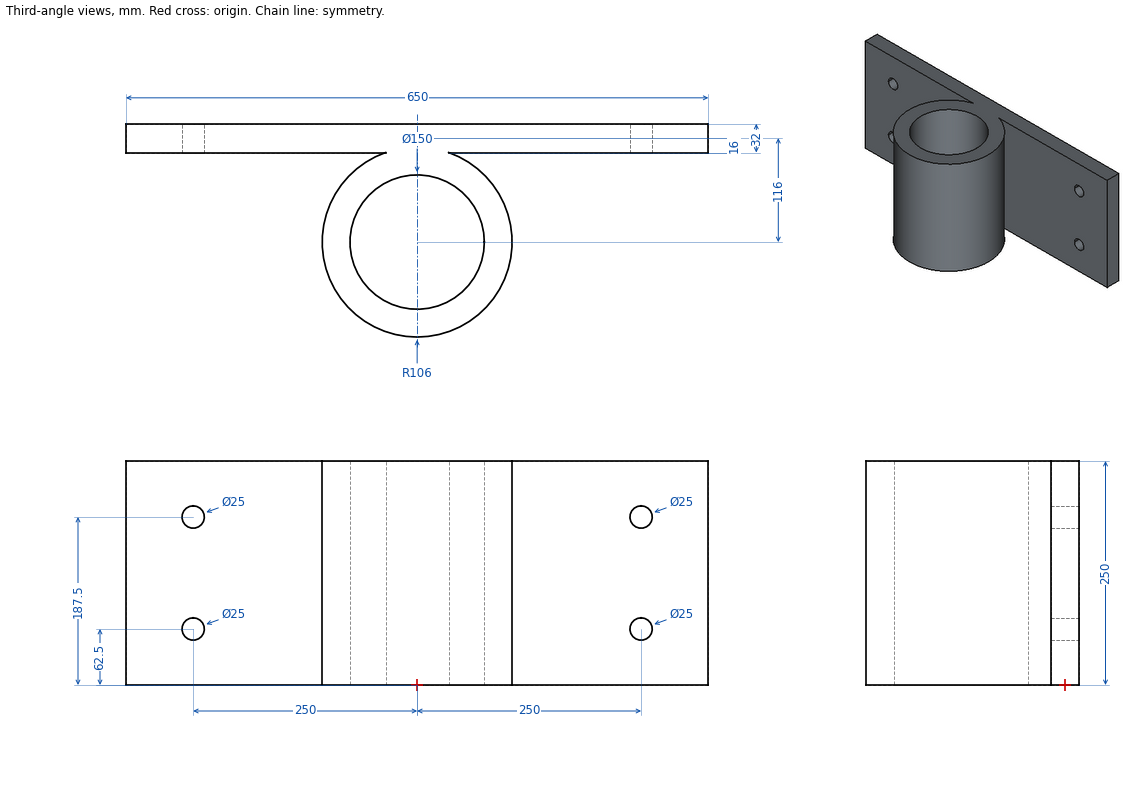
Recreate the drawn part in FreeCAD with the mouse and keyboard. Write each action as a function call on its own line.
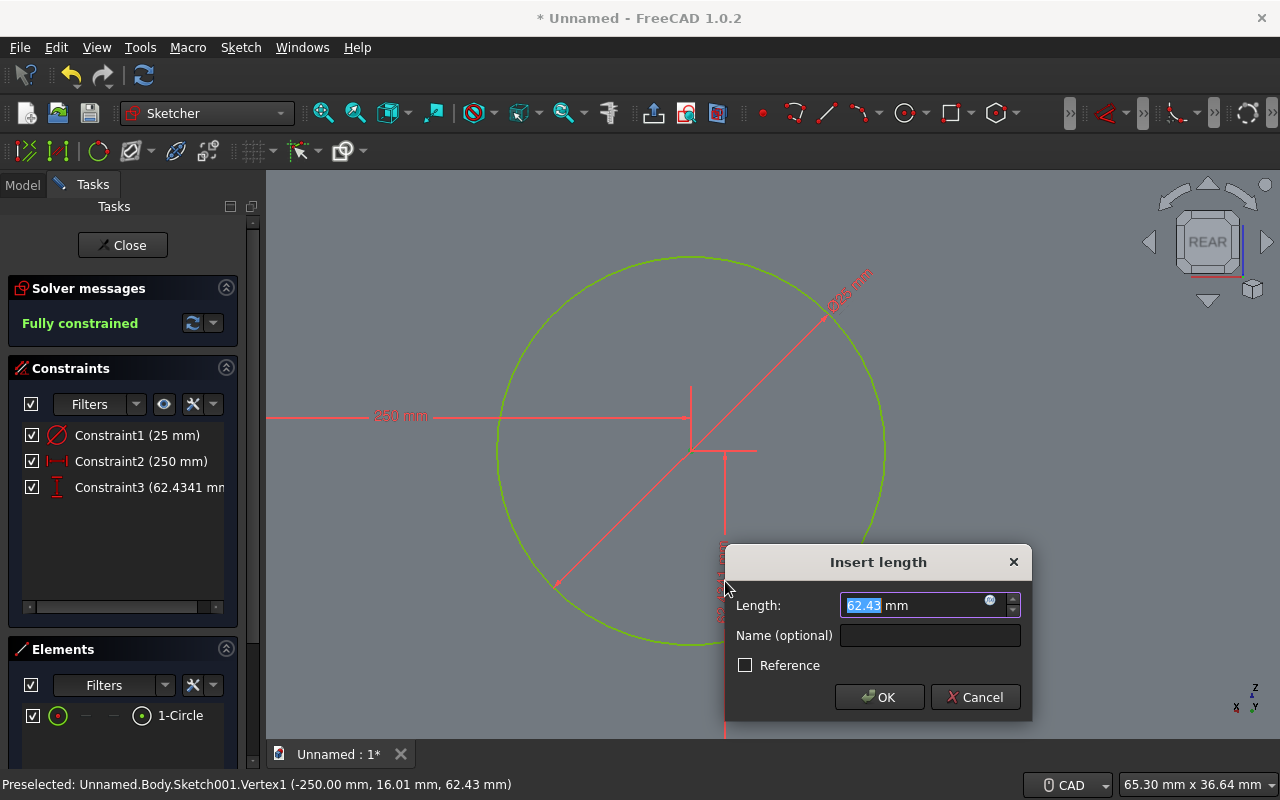
text(62.5)
key(Return)
key(Escape)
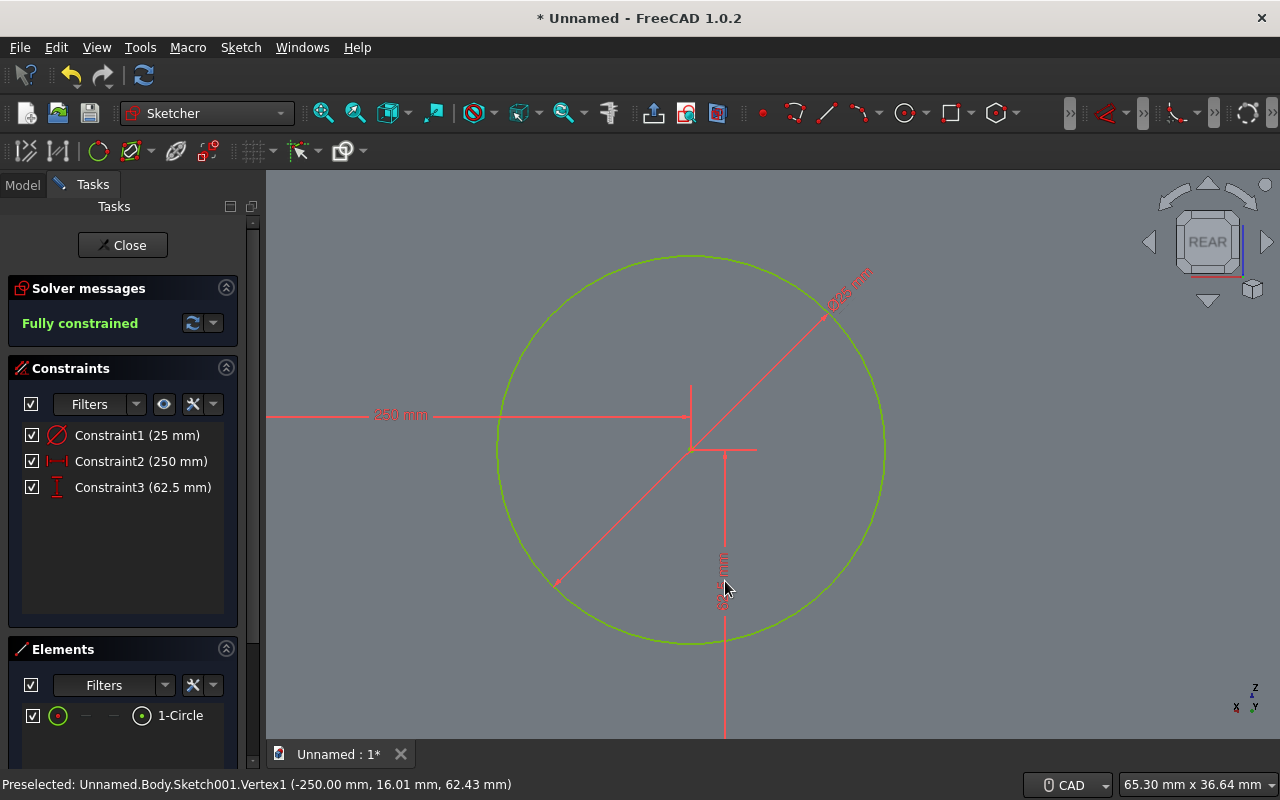
click(123, 245)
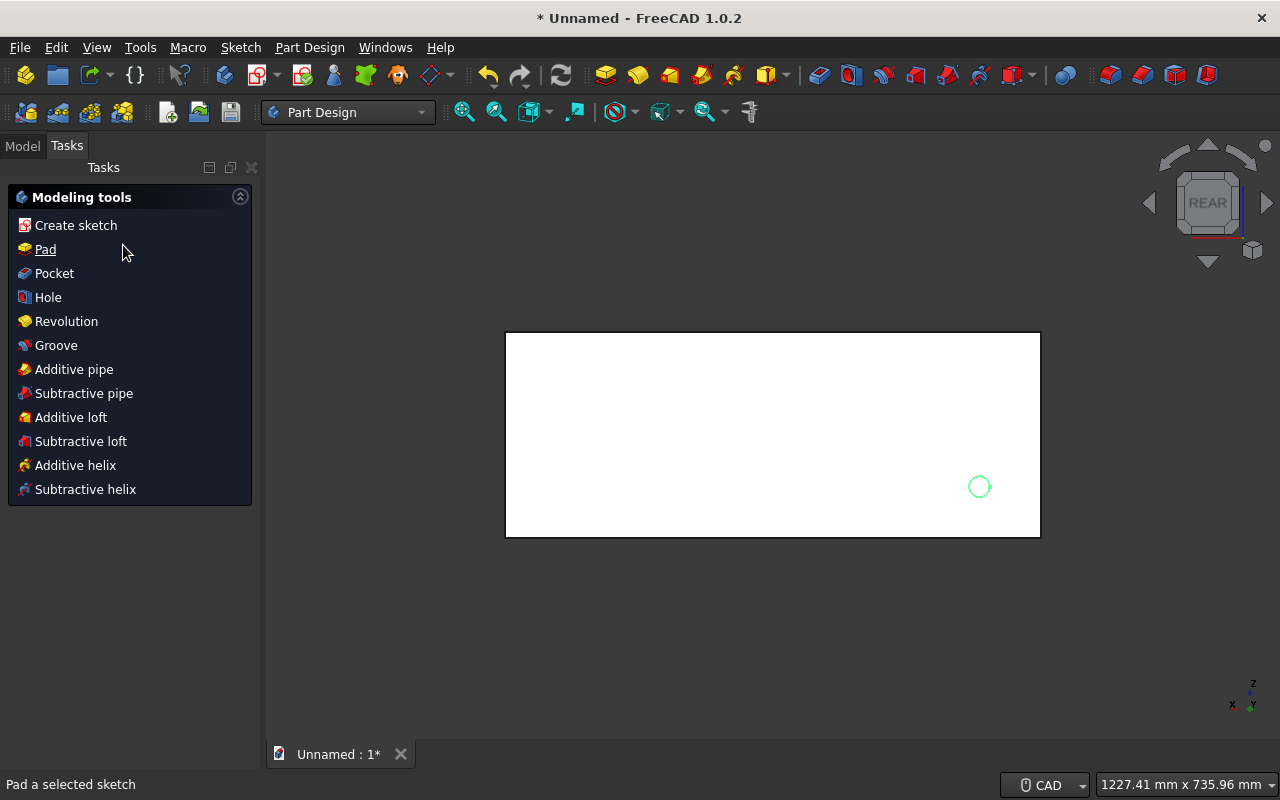
click(820, 76)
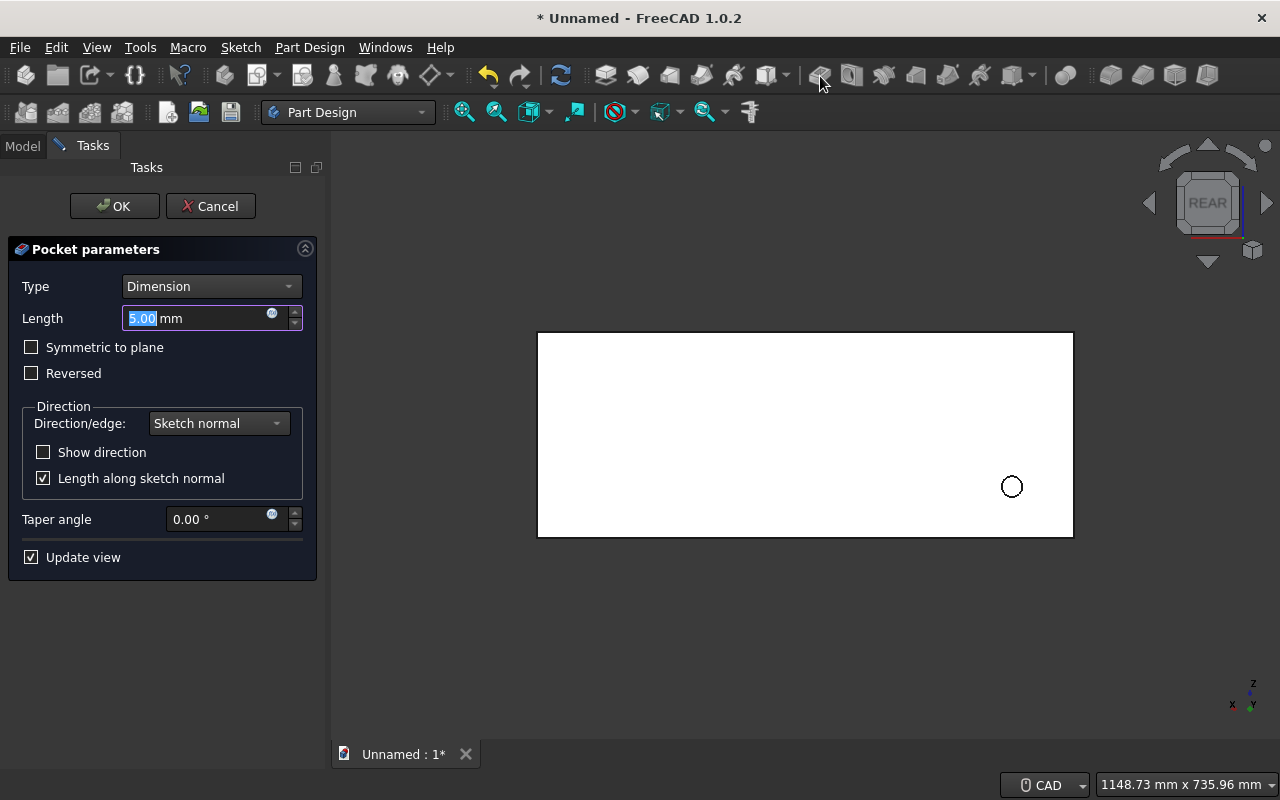
click(212, 286)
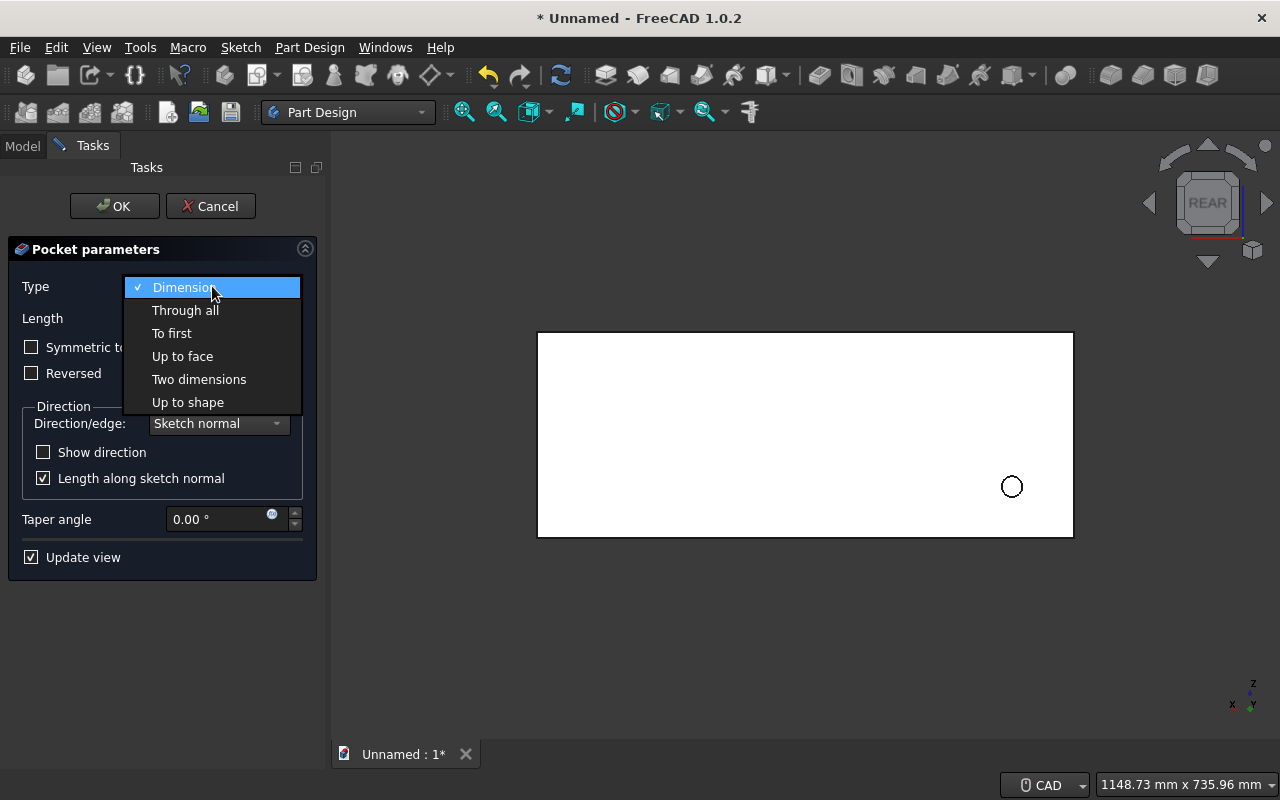
click(212, 334)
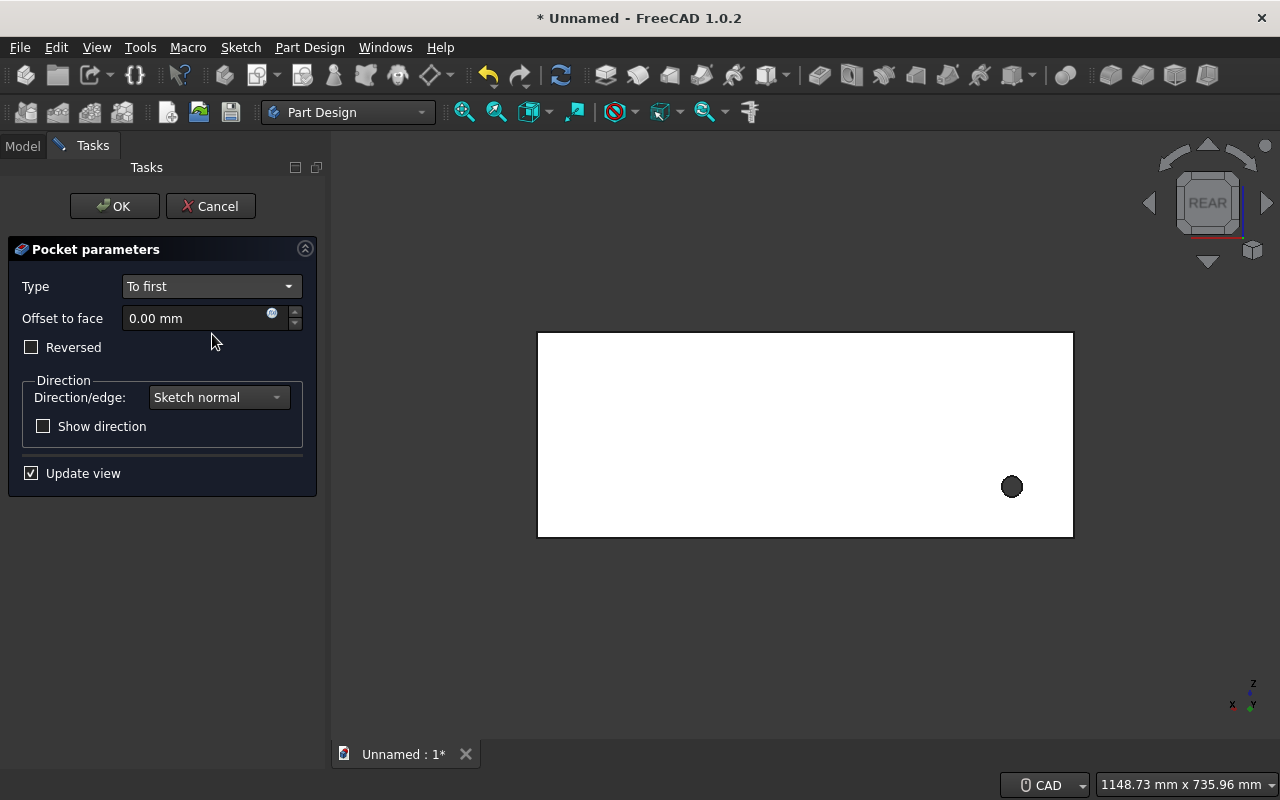
click(115, 206)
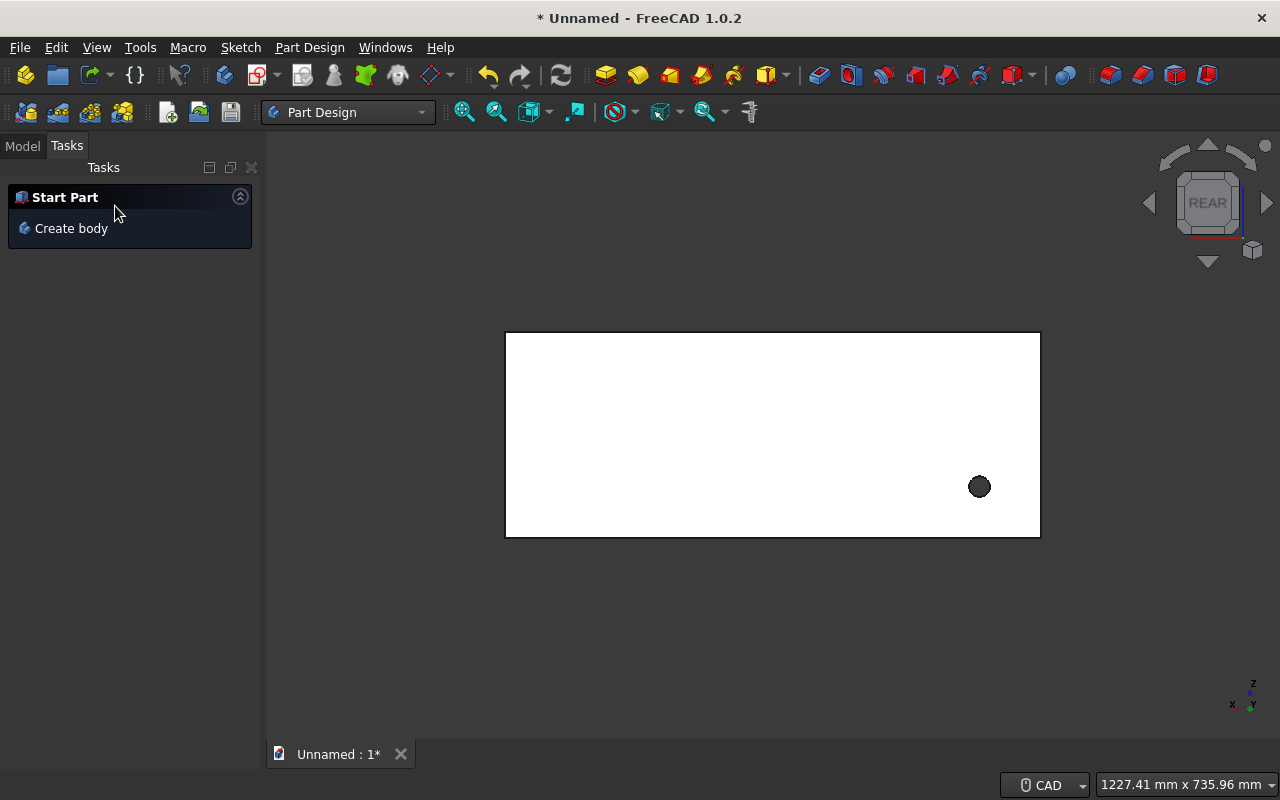
click(620, 434)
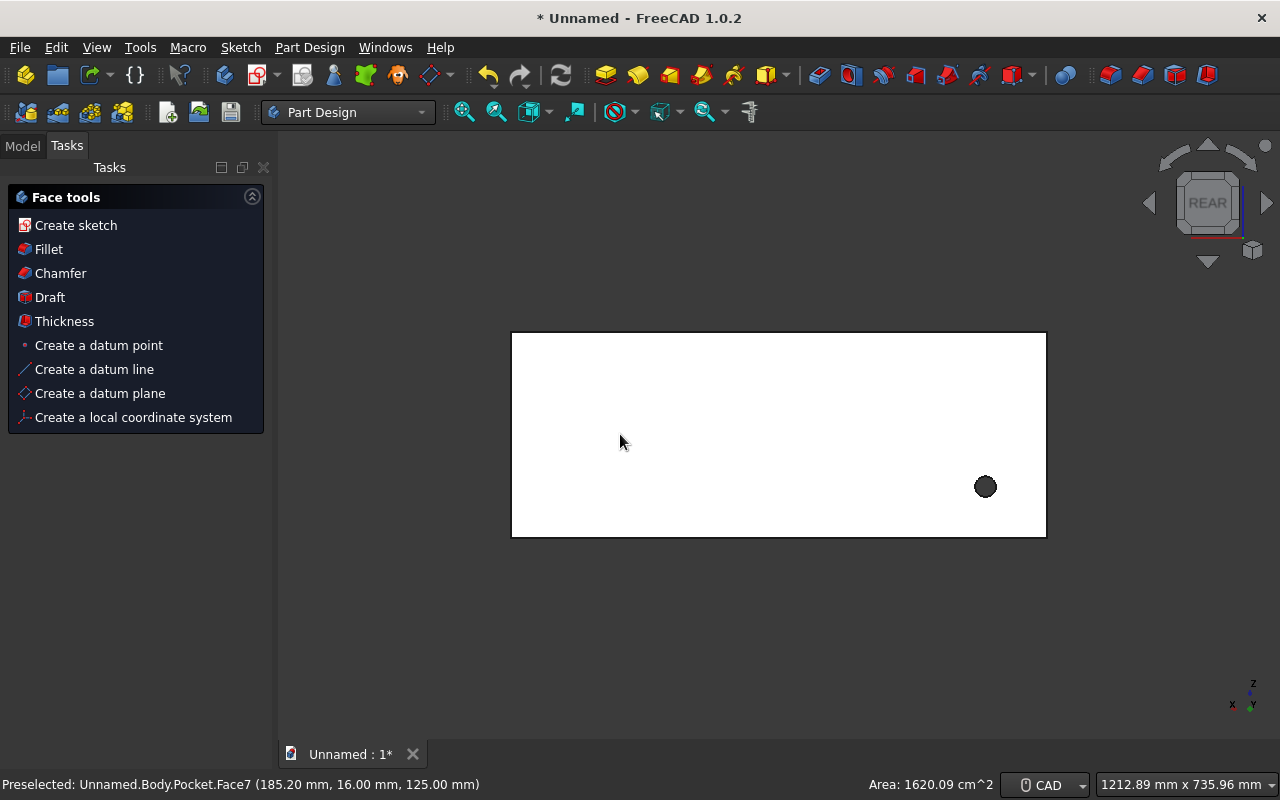
click(258, 76)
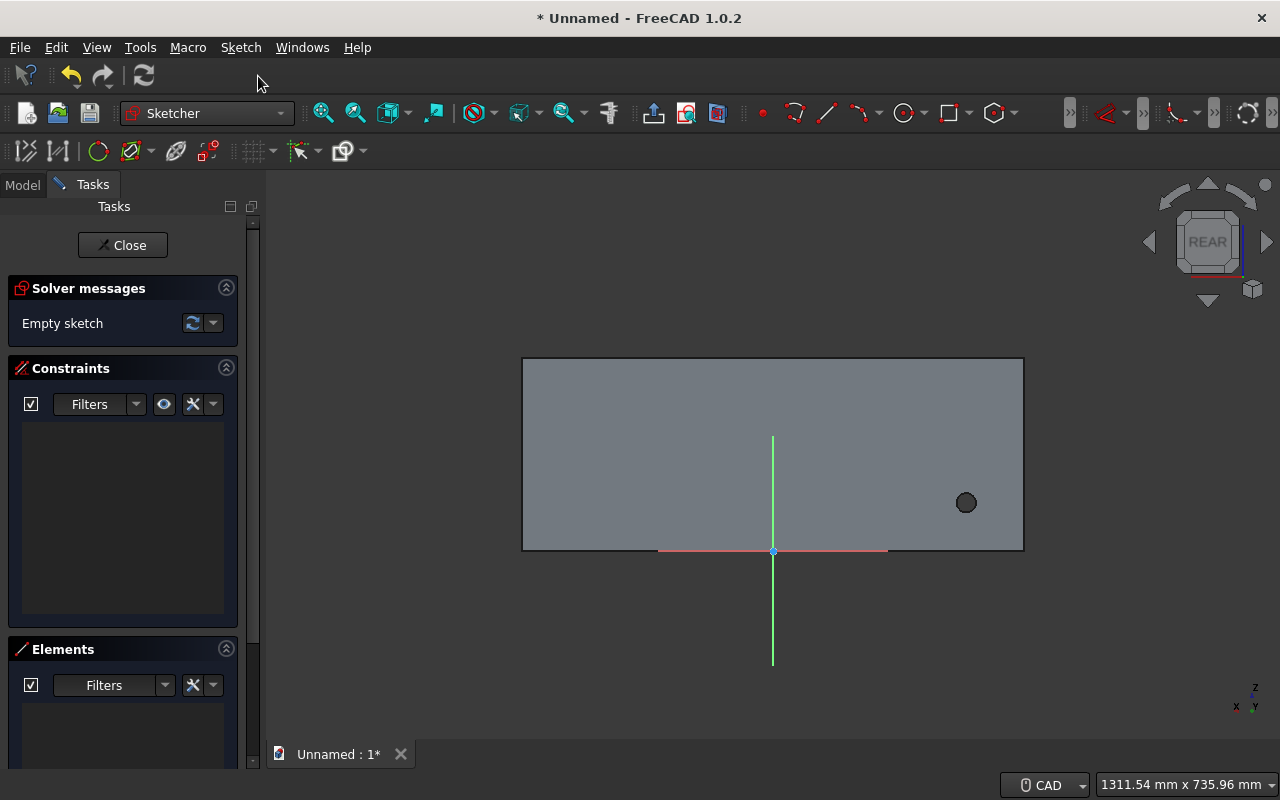
scroll(573, 505, up, 15)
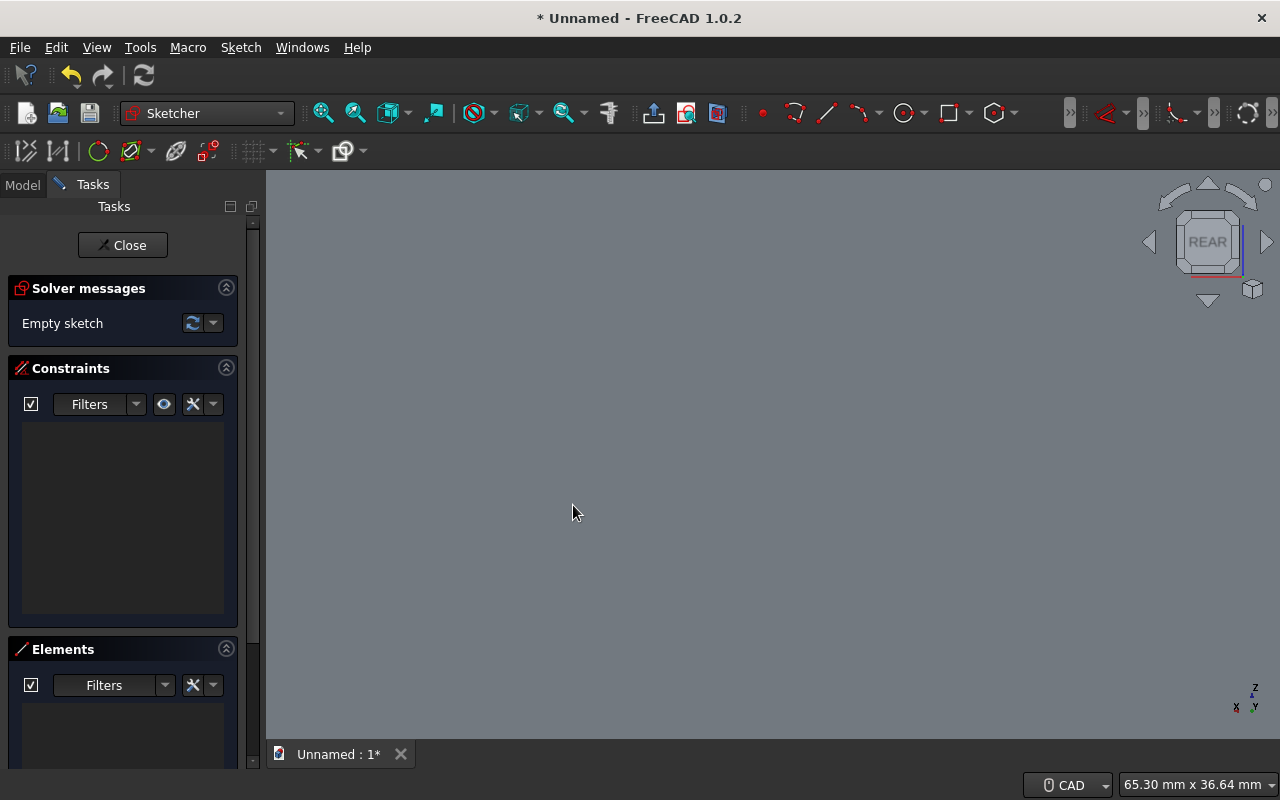
click(904, 114)